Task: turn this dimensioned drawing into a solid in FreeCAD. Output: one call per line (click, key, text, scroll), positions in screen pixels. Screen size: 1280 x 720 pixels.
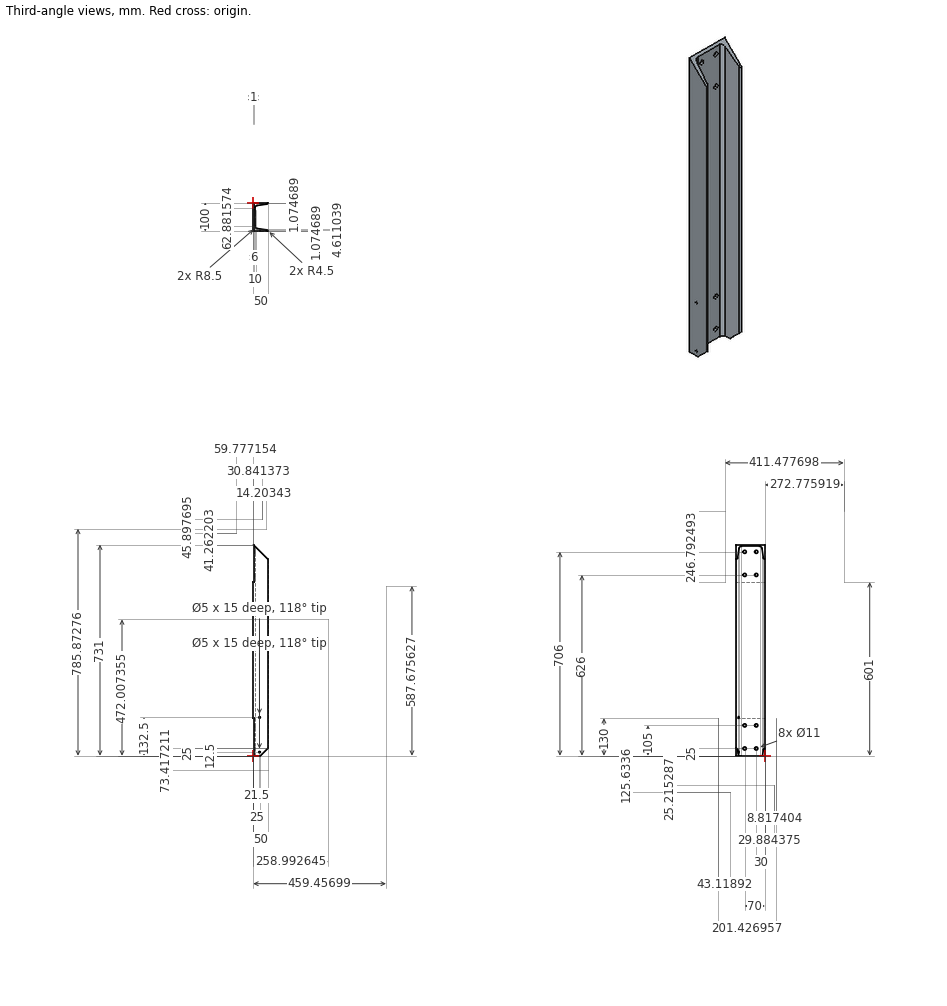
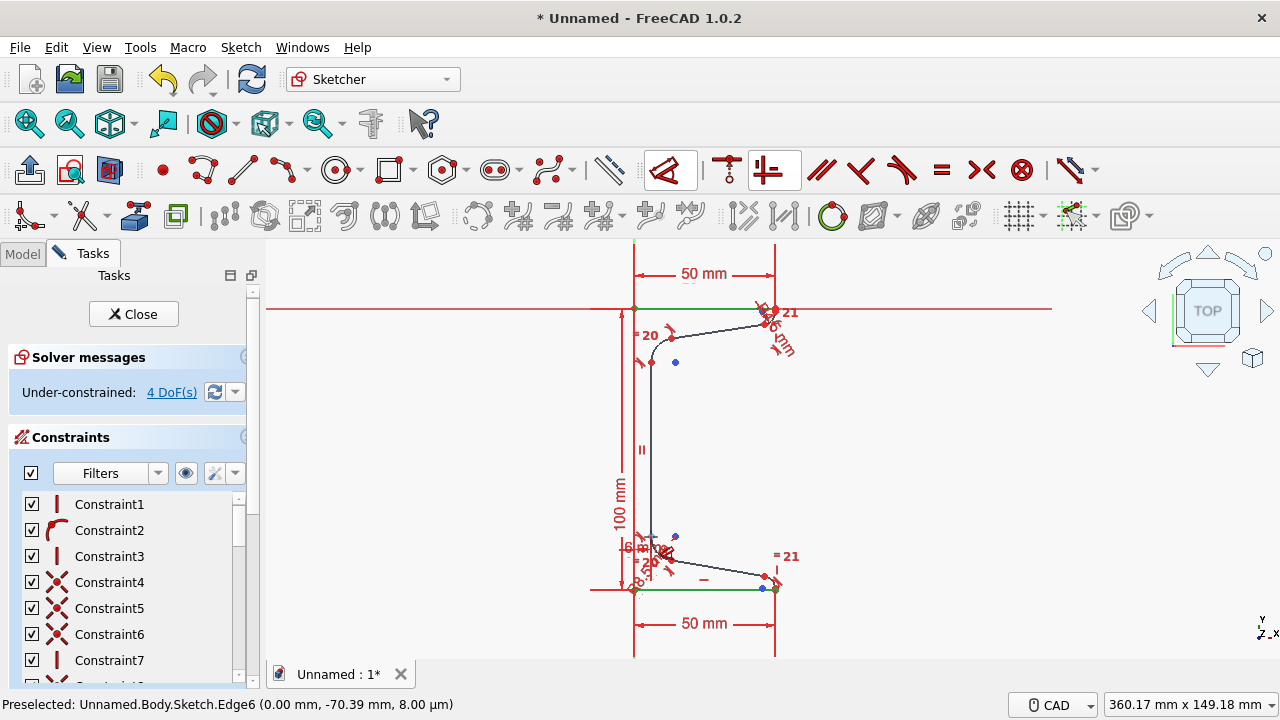
scroll(775, 310, up, 13)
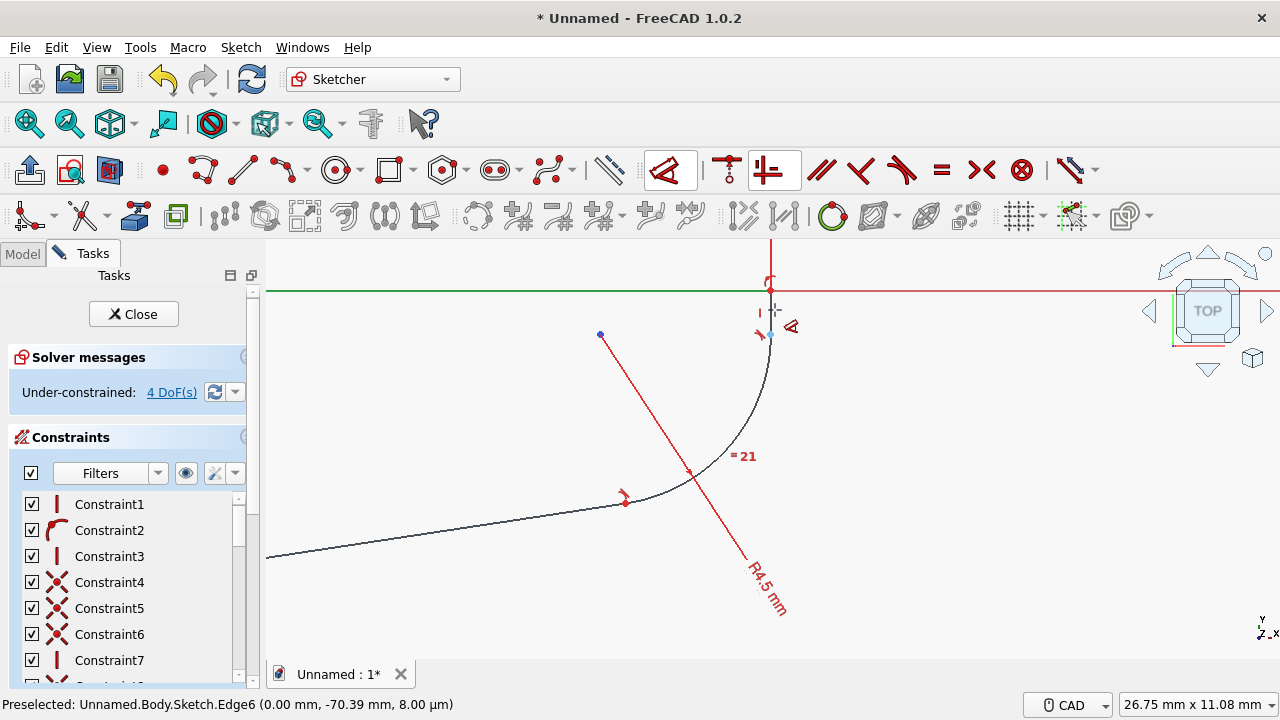
click(771, 313)
click(805, 313)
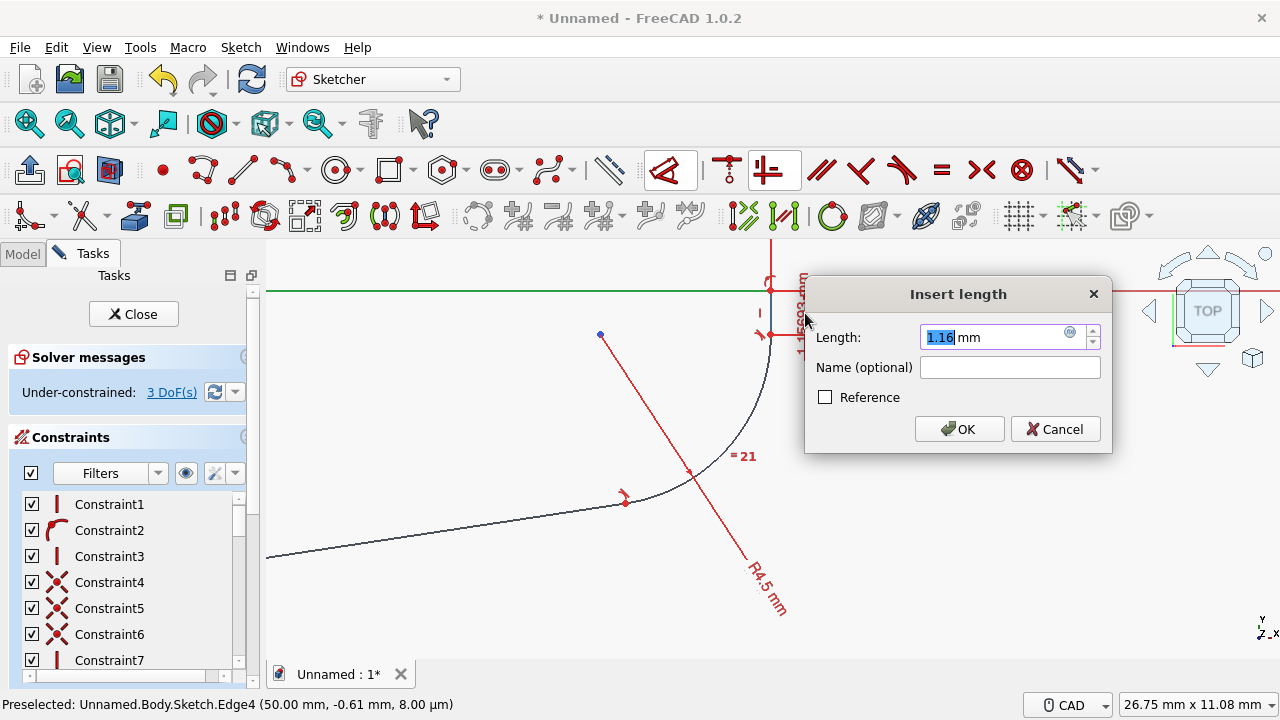
text(1.074689)
key(Return)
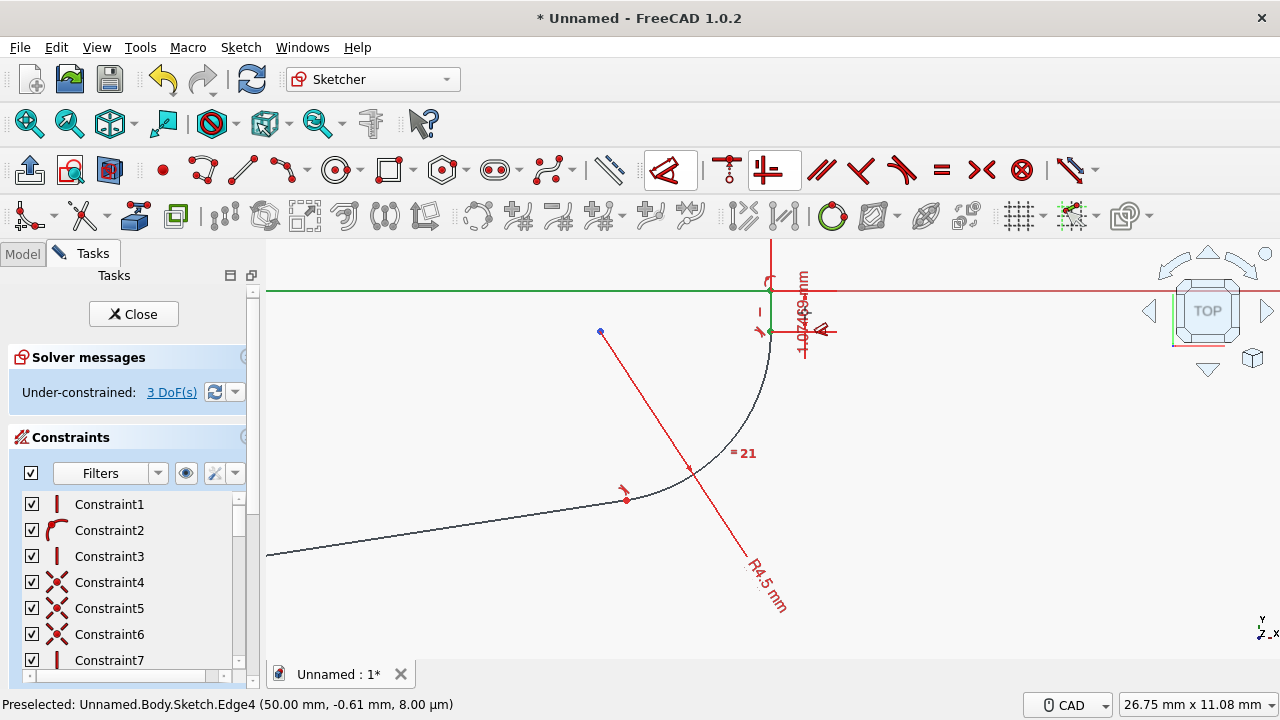
scroll(775, 310, down, 13)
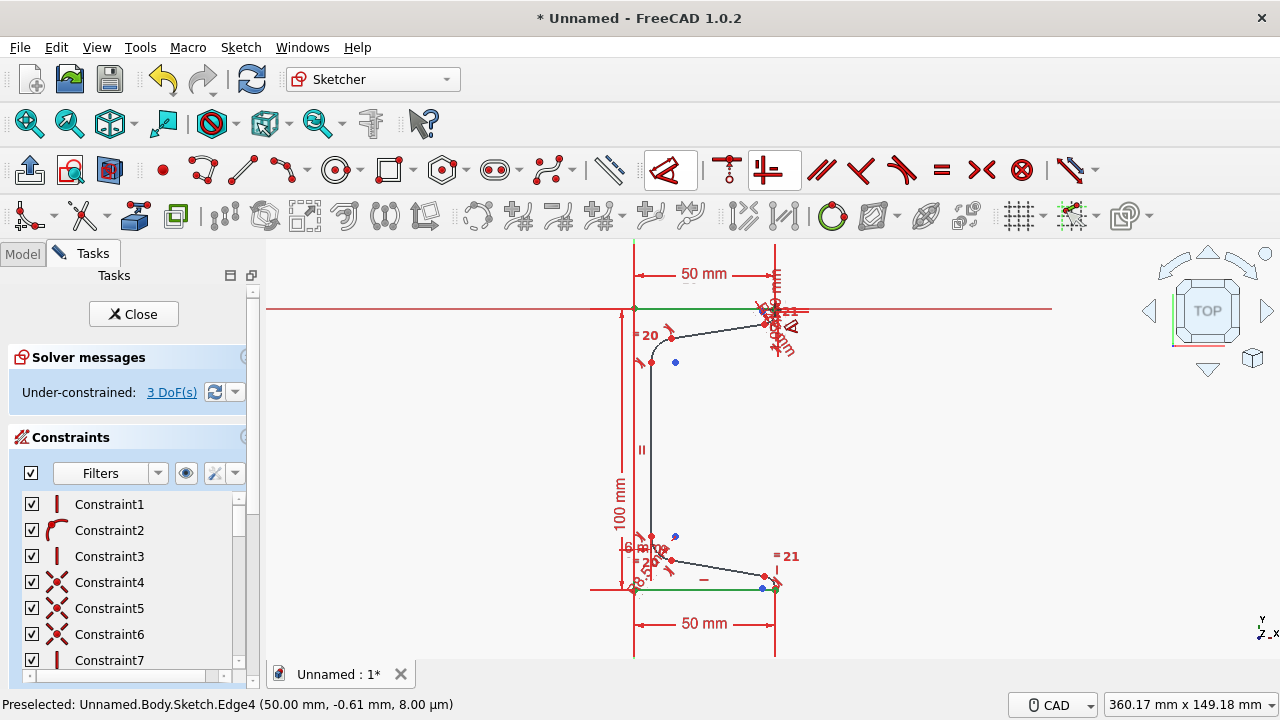
scroll(775, 590, up, 13)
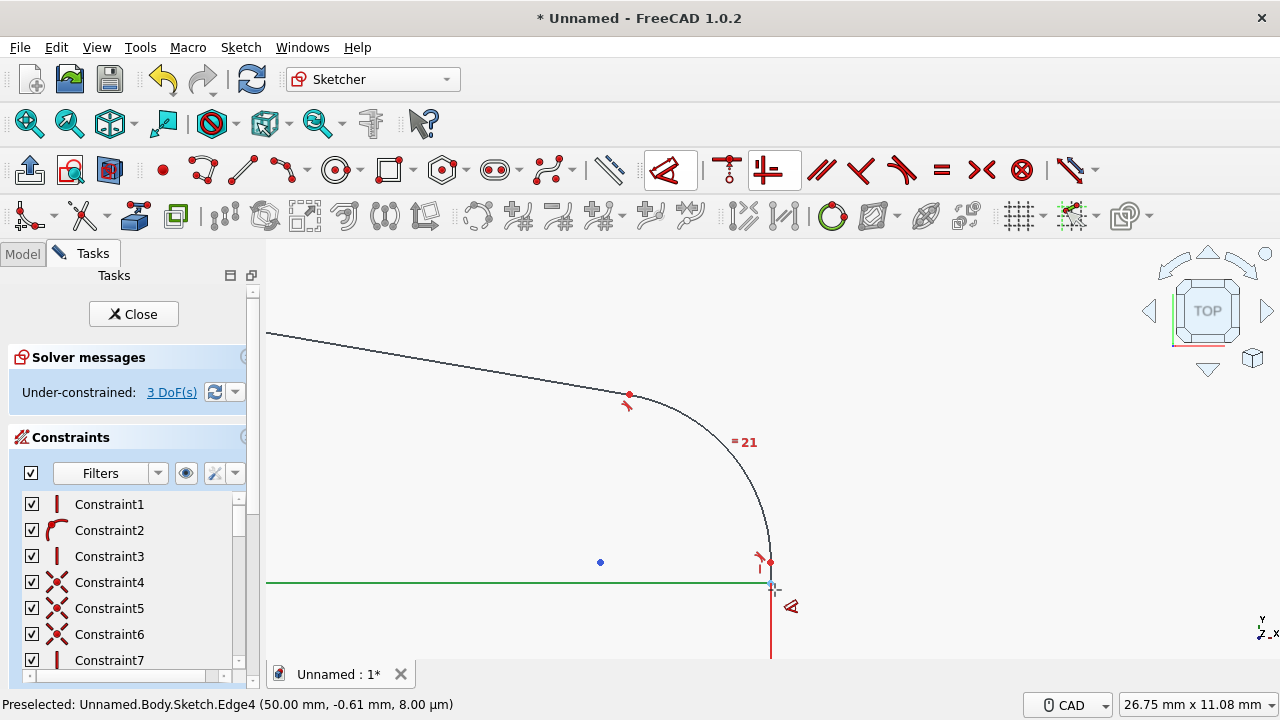
click(771, 573)
click(805, 573)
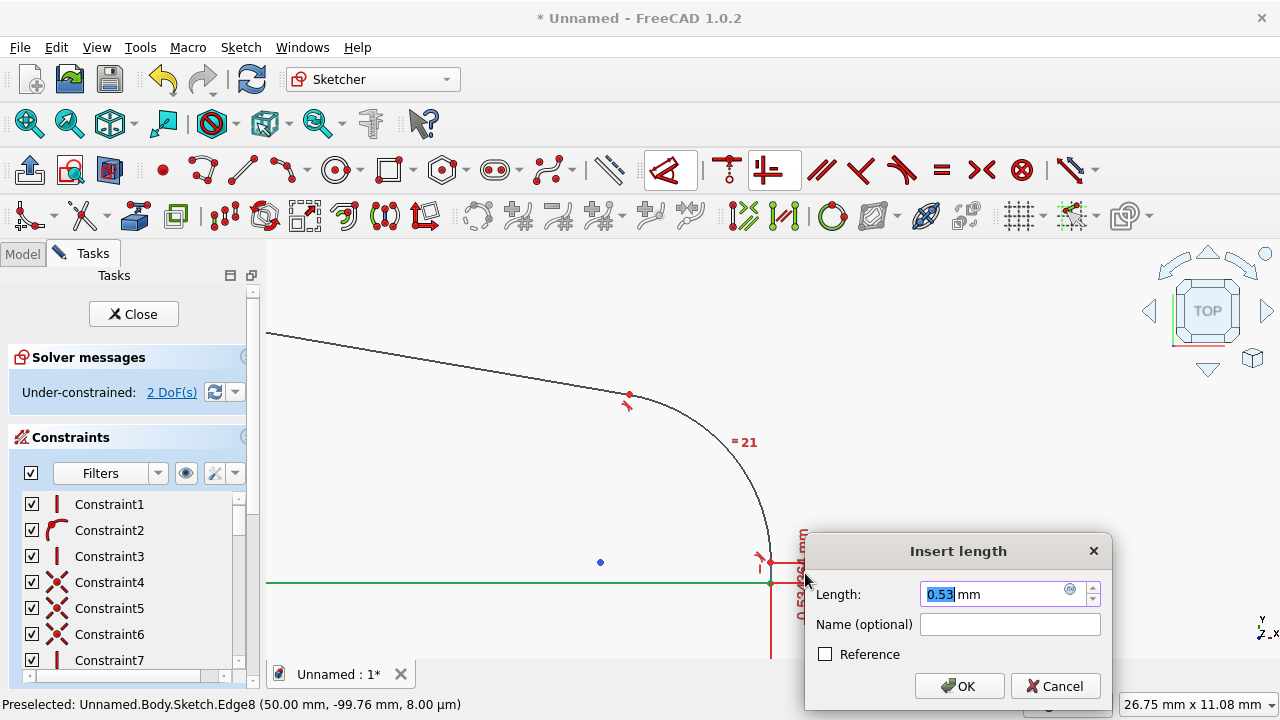
text(1.074689)
key(Return)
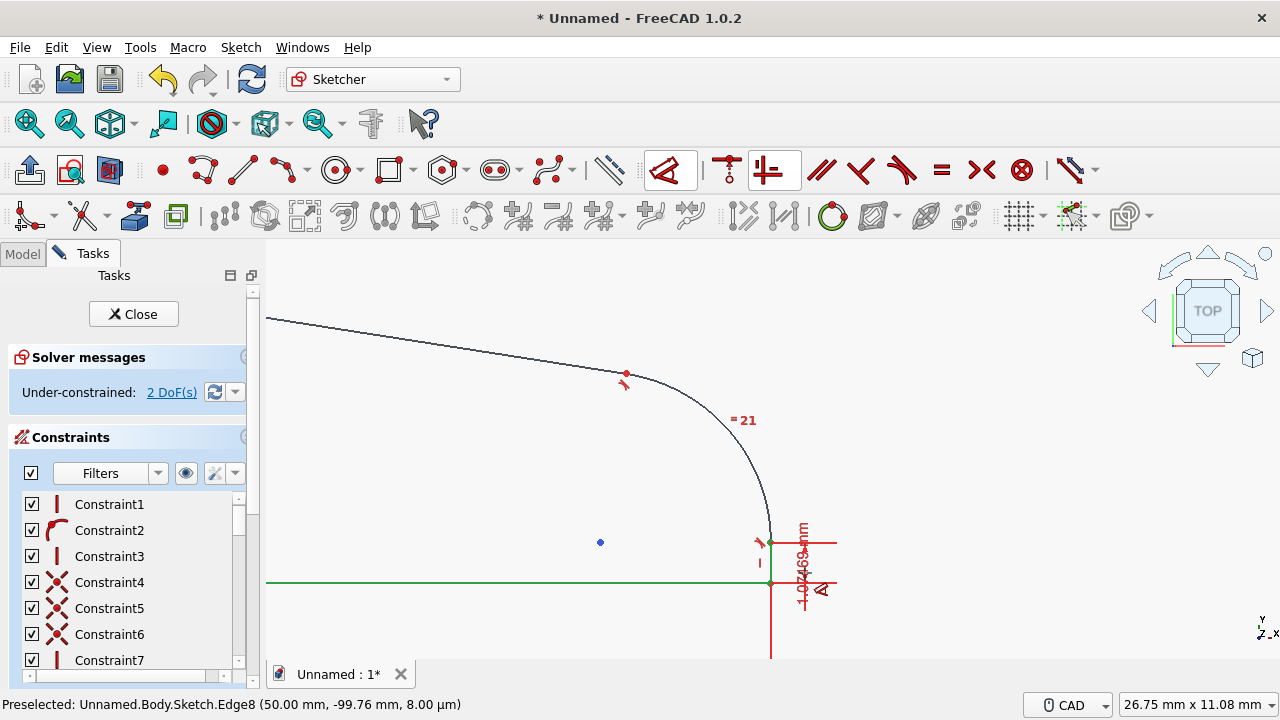
scroll(775, 590, down, 13)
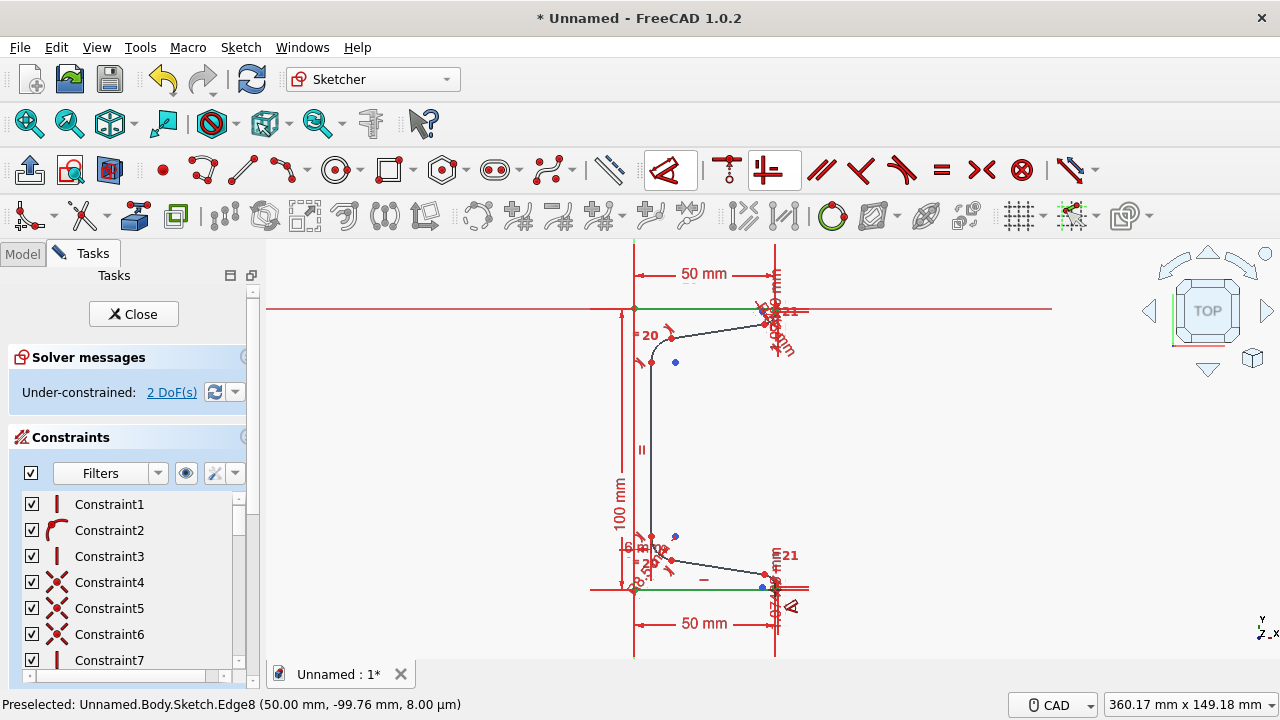
click(651, 484)
click(617, 449)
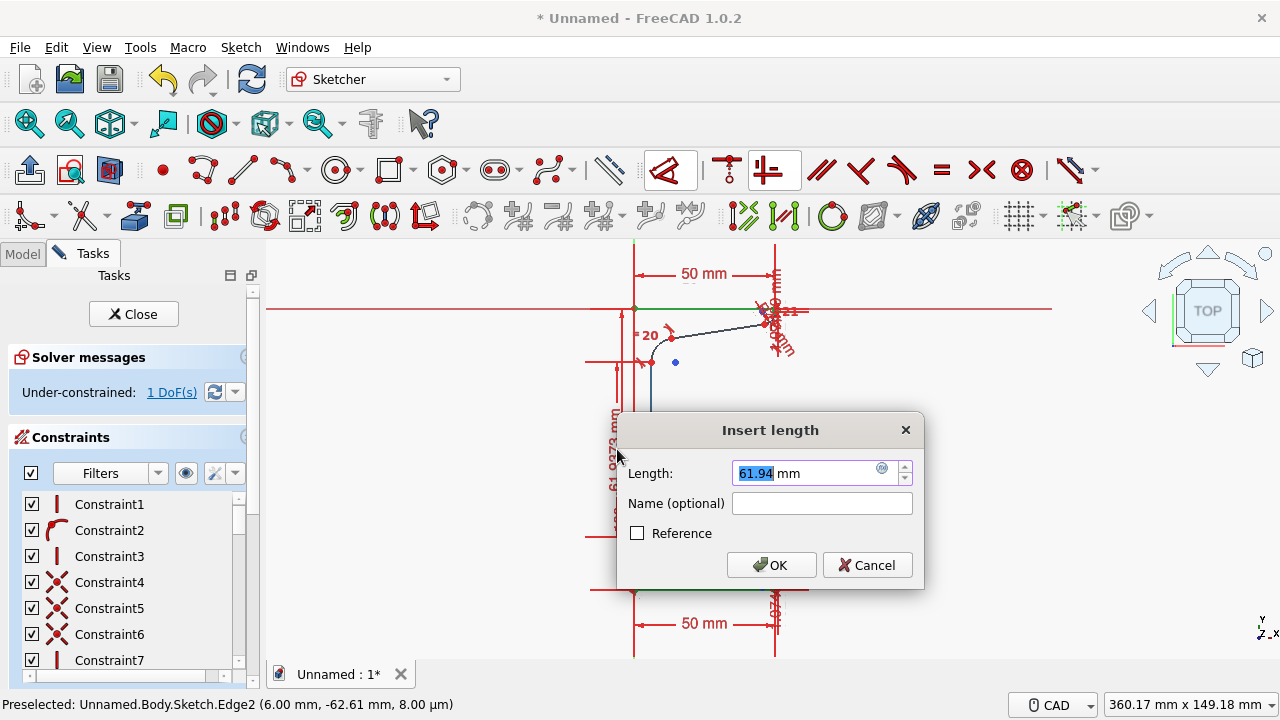
text(62.881574)
key(Return)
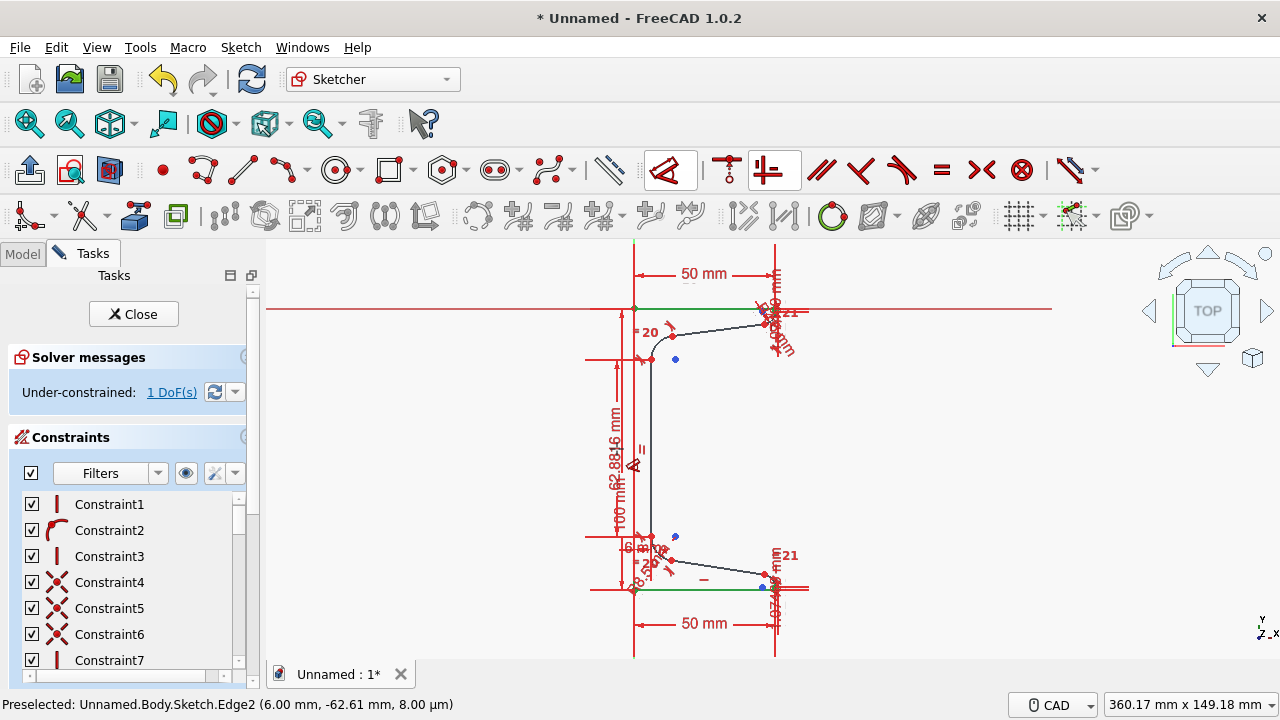
scroll(737, 570, up, 6)